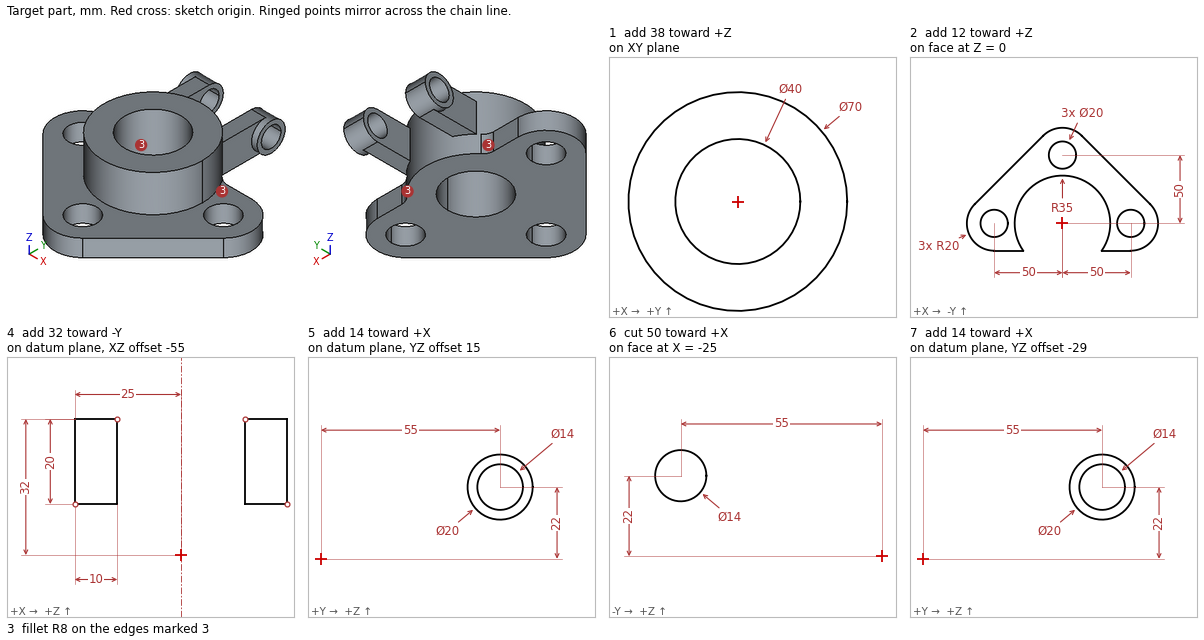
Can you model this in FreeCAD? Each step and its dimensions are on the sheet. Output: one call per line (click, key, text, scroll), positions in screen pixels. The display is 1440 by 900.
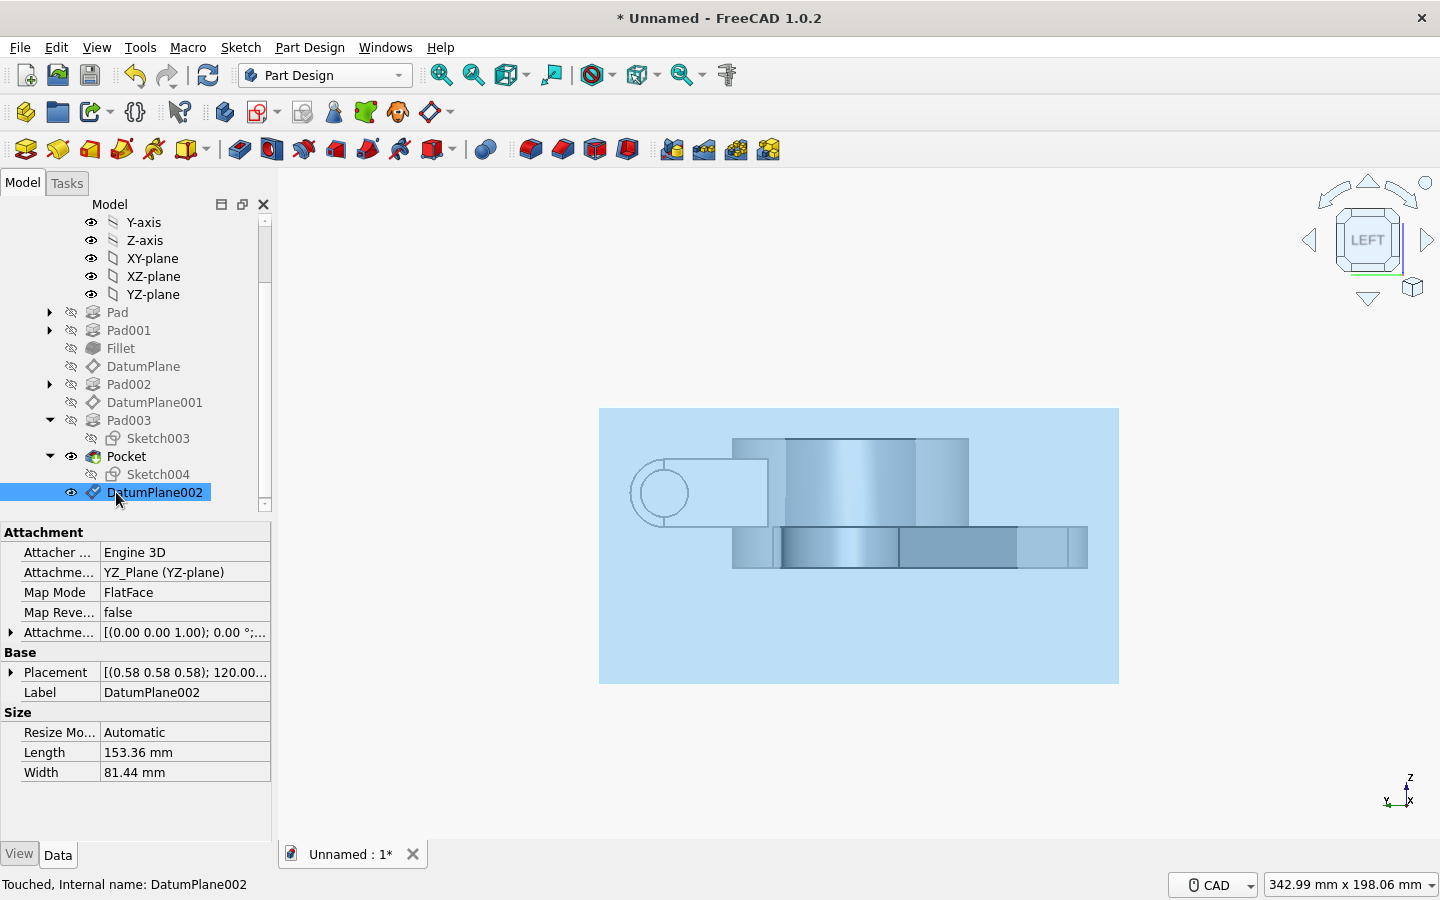
click(258, 112)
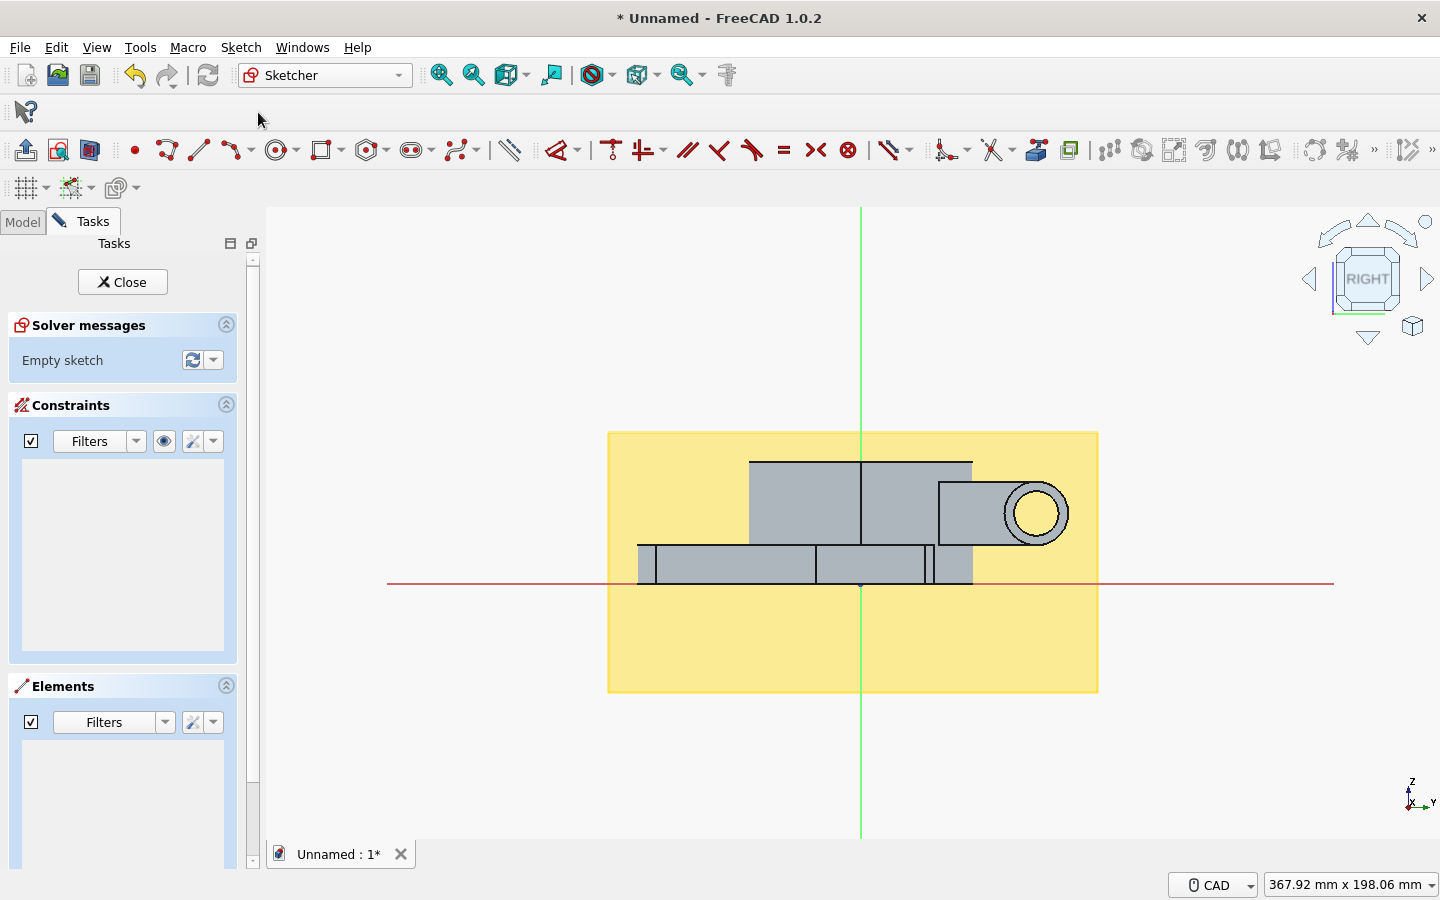
key(q)
key(s)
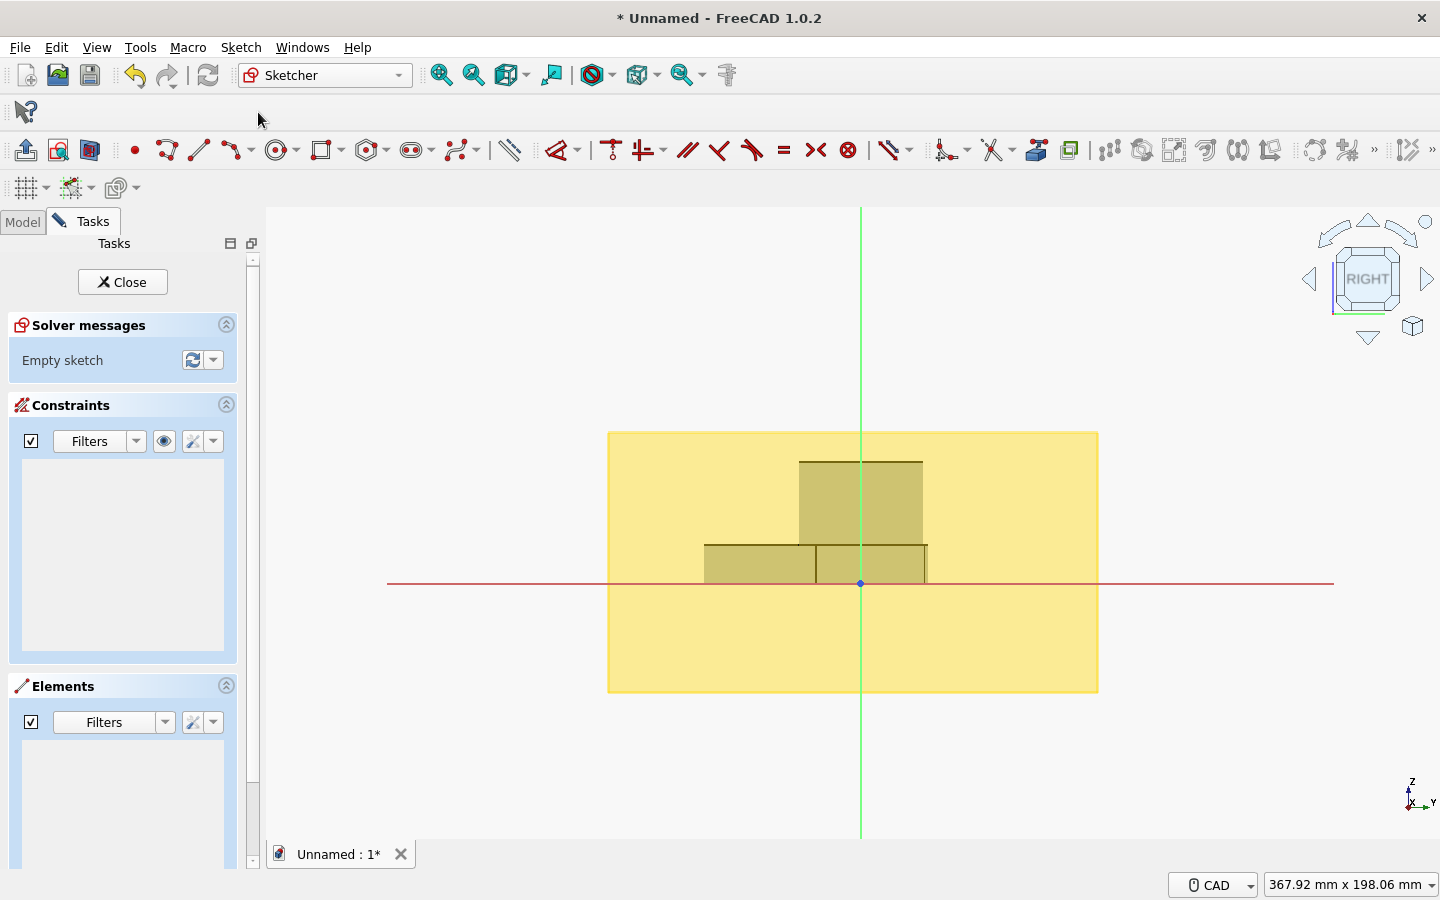
scroll(1086, 512, up, 9)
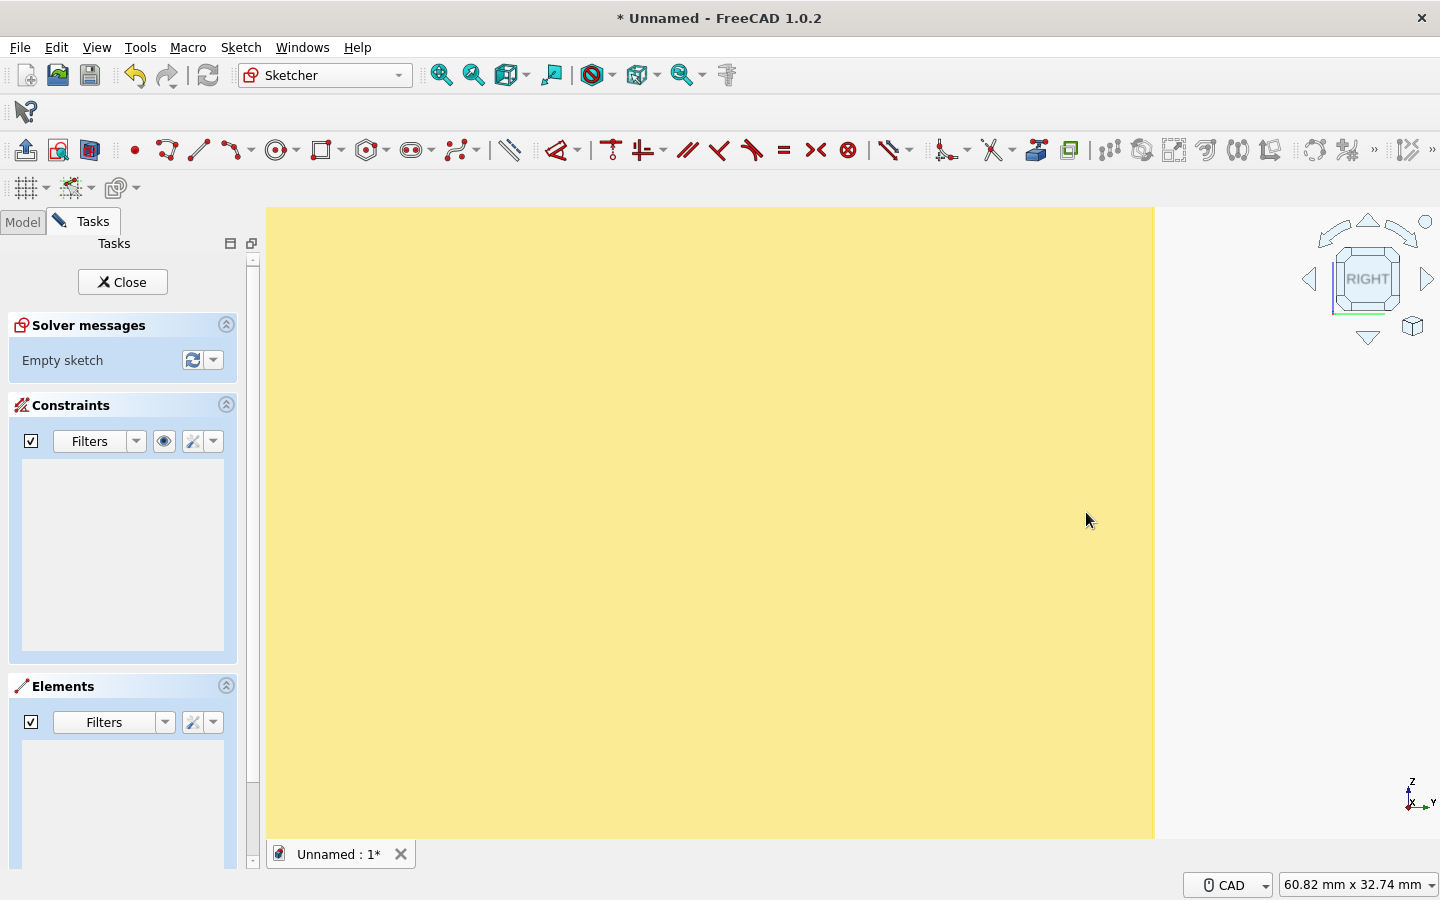
click(276, 150)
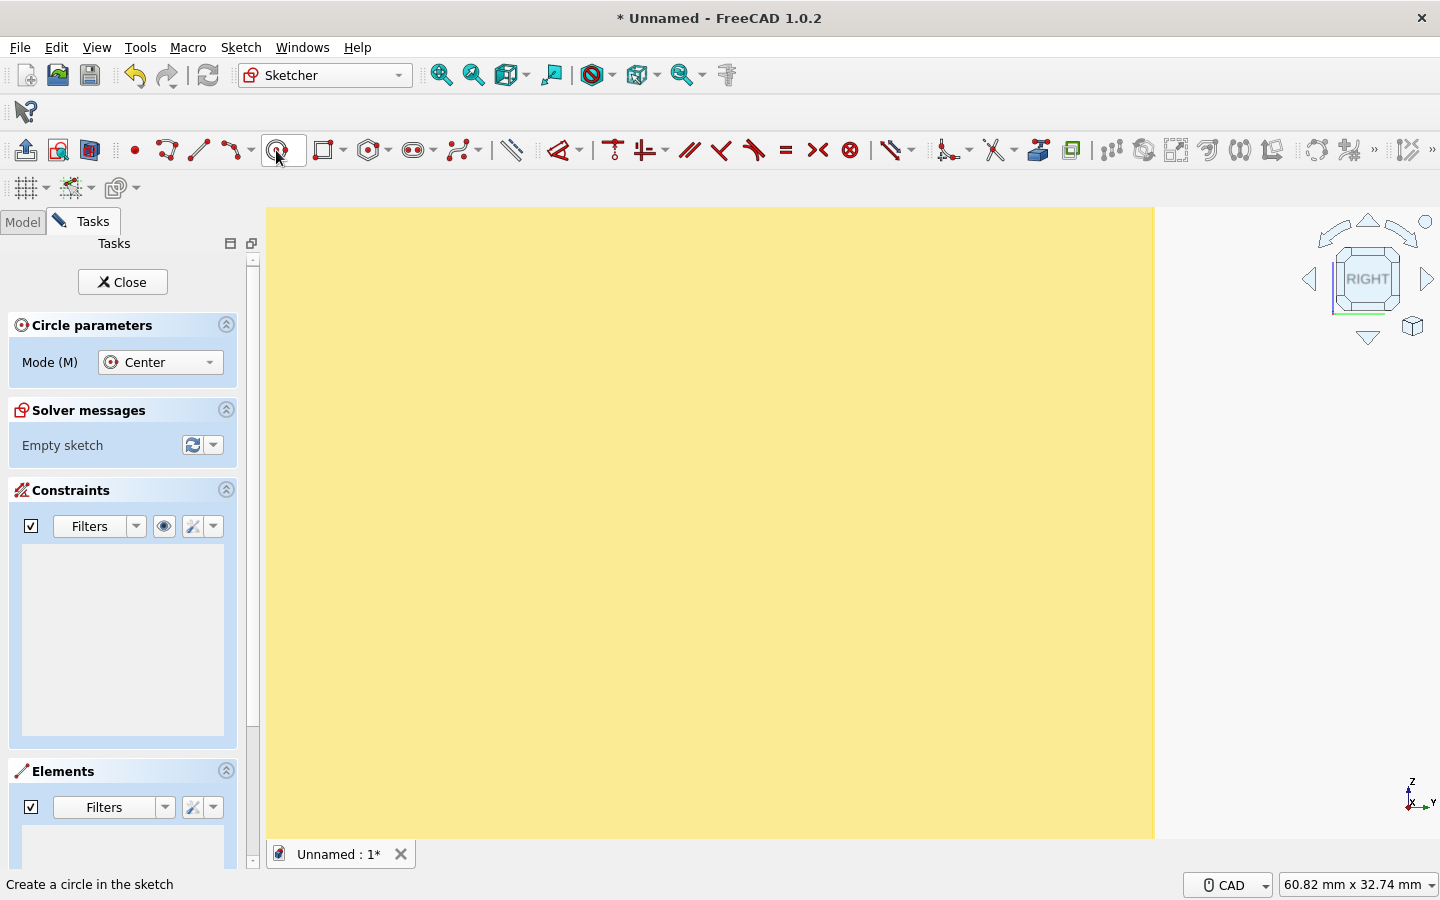
click(782, 518)
click(919, 382)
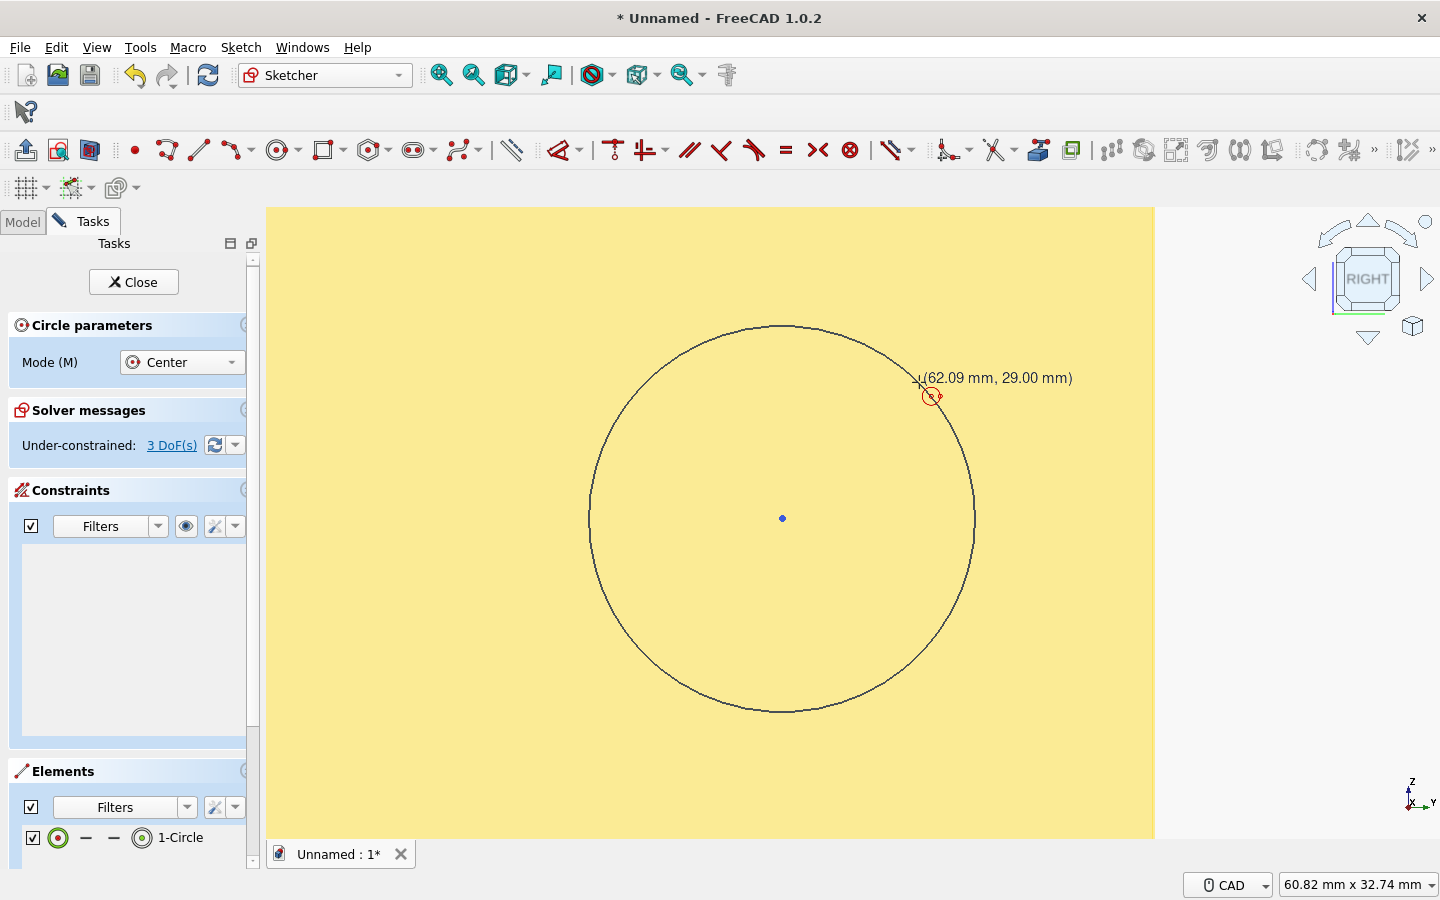
click(782, 519)
click(878, 423)
key(Escape)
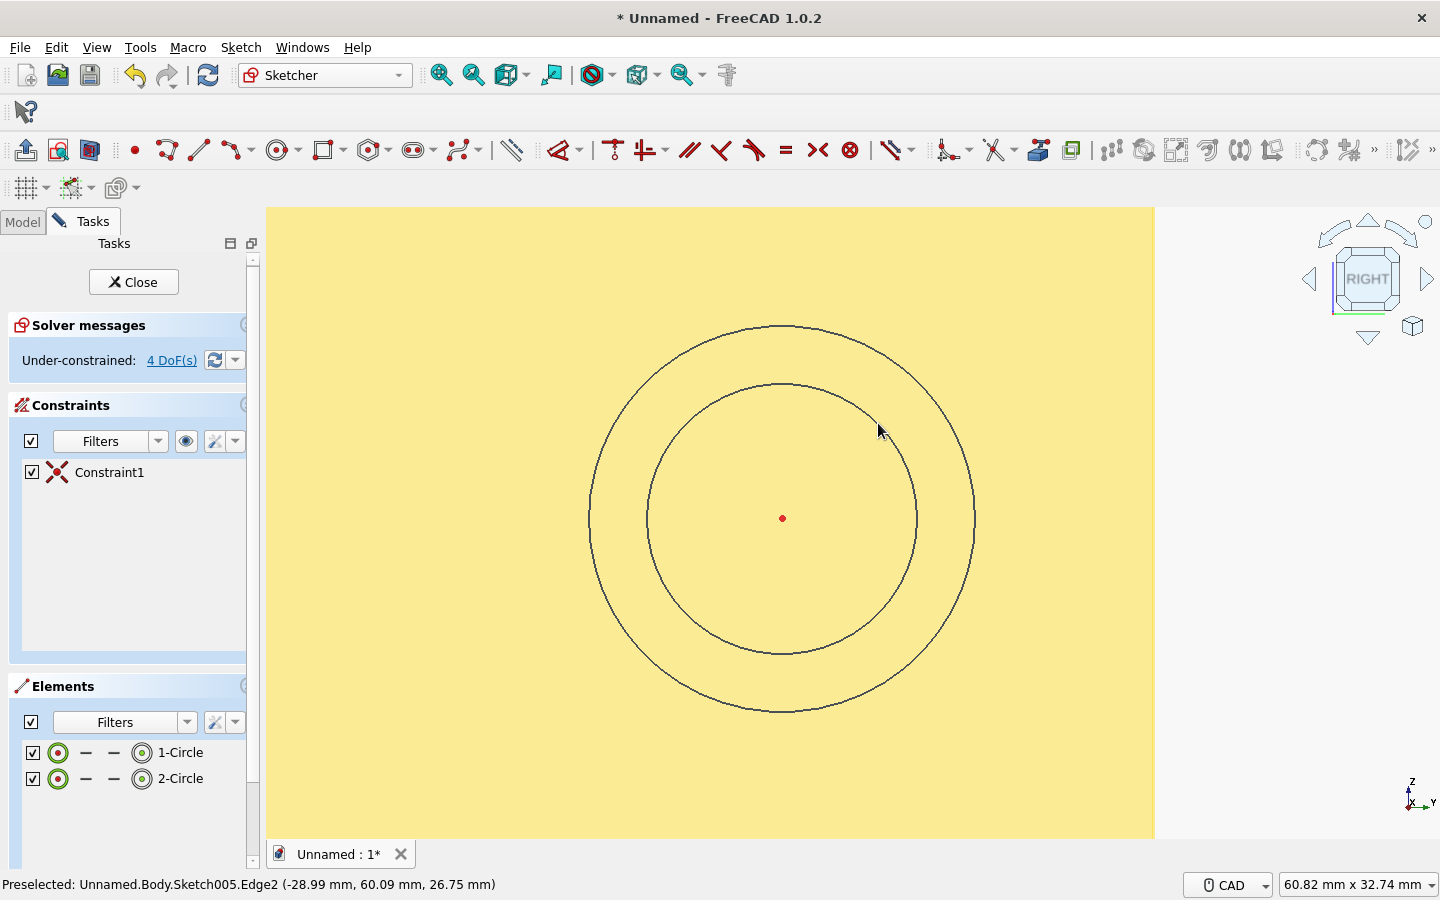
key(d)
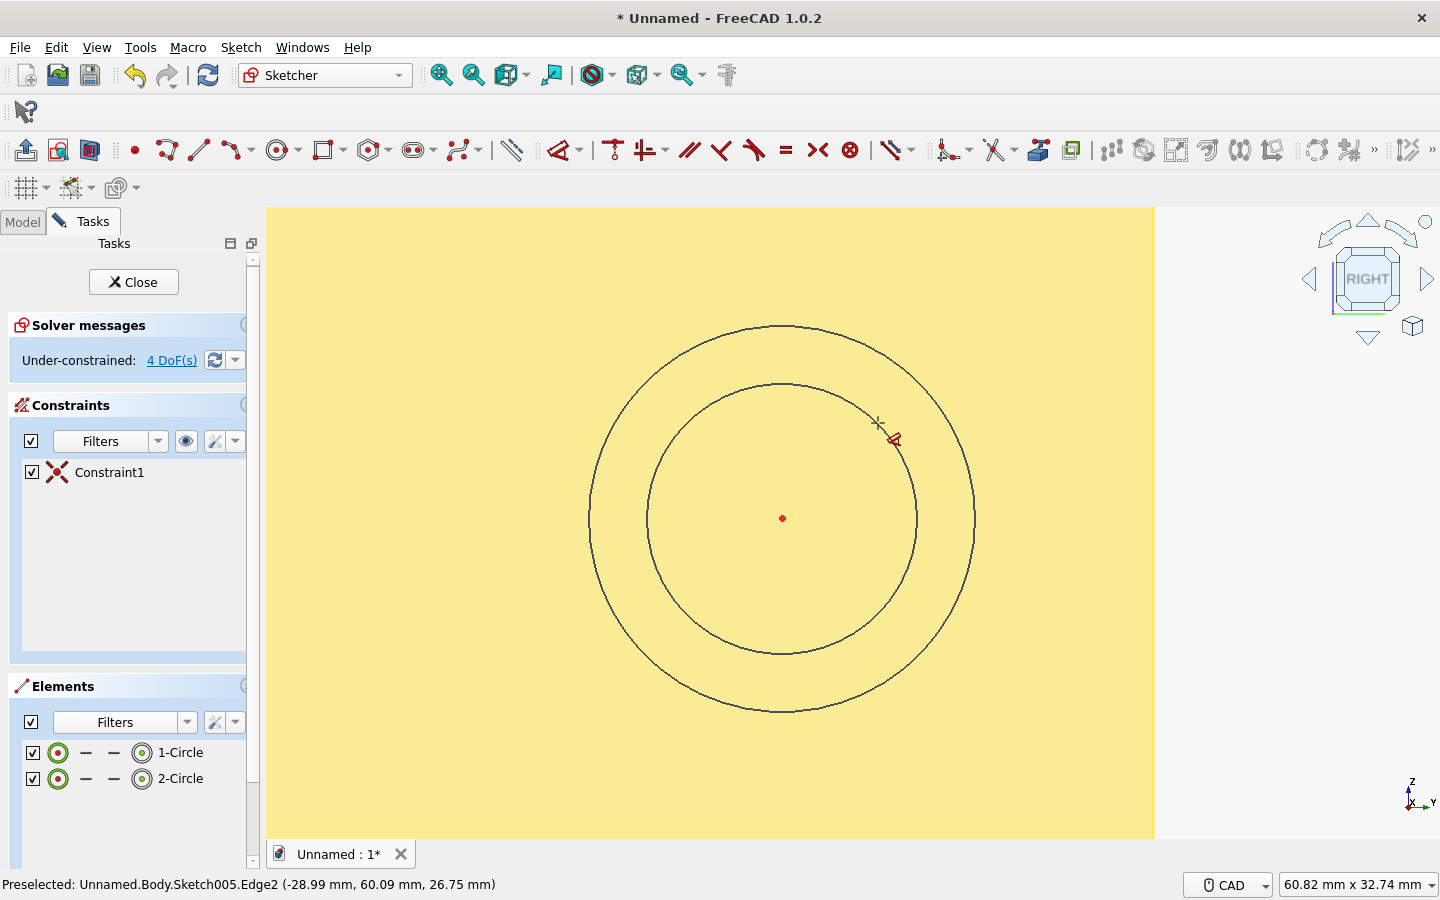
click(918, 382)
click(941, 359)